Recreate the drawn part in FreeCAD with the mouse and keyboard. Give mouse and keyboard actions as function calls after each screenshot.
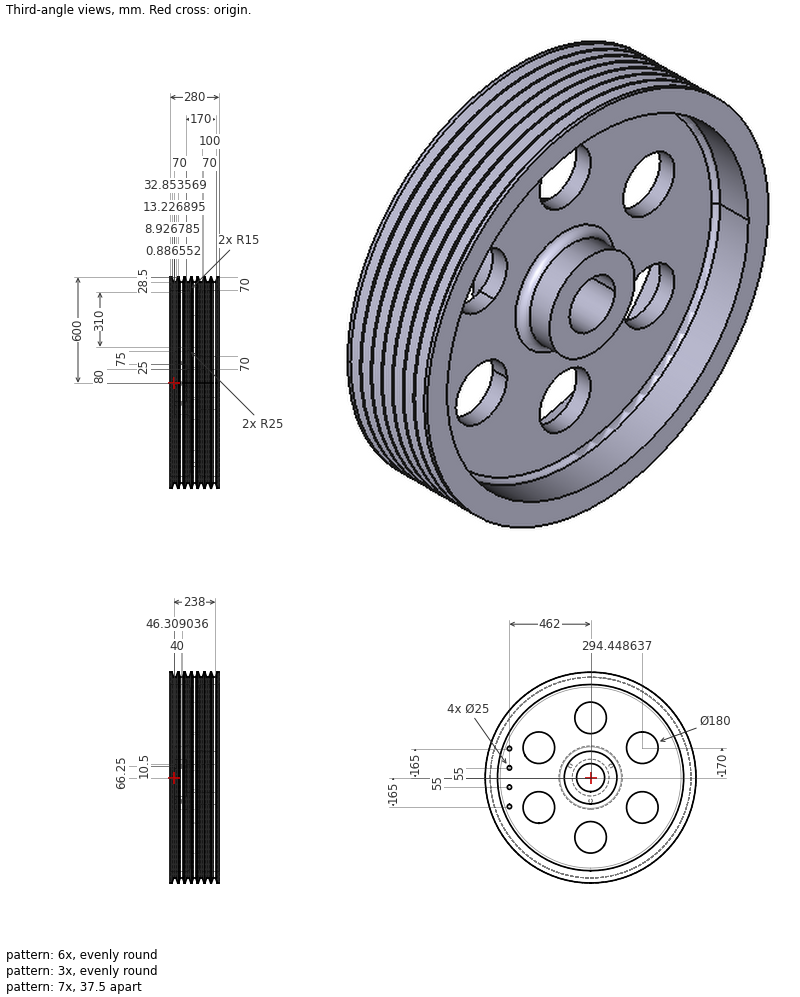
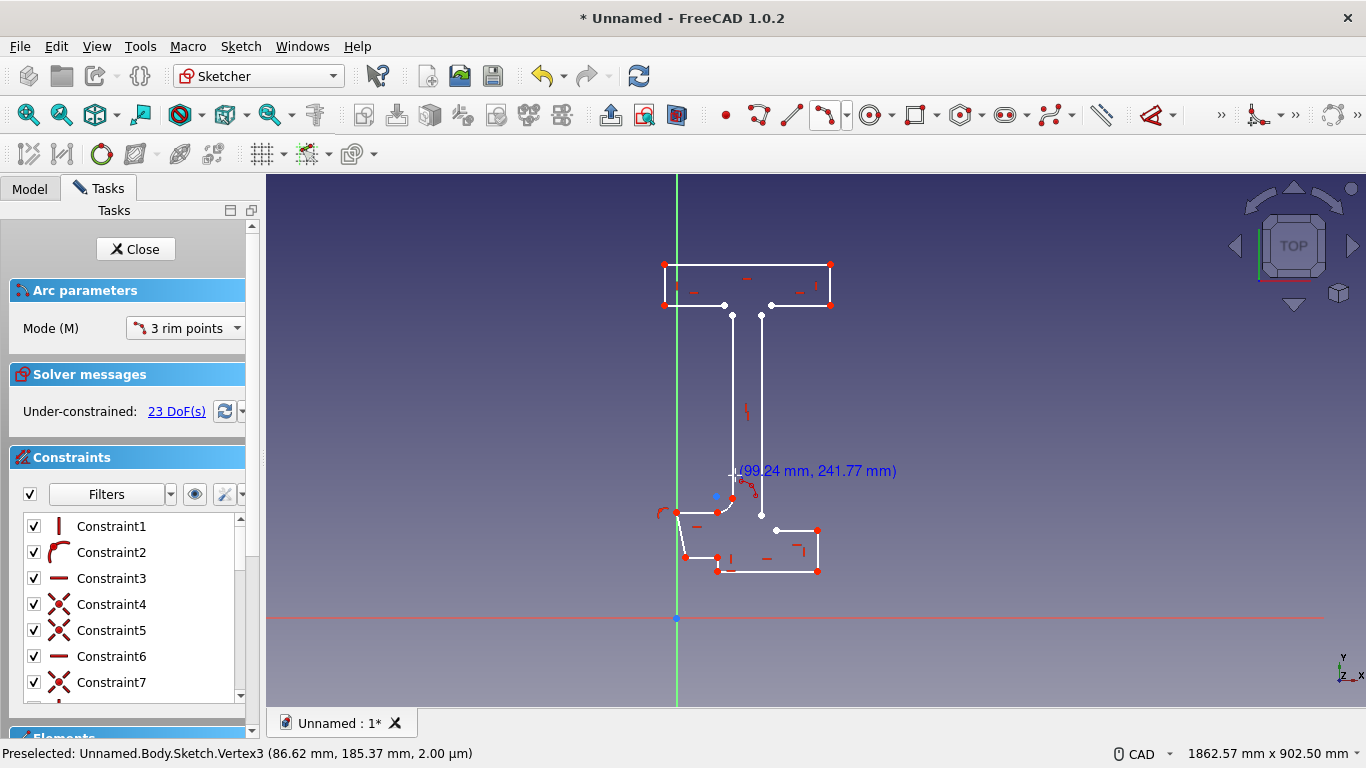
click(777, 531)
click(762, 516)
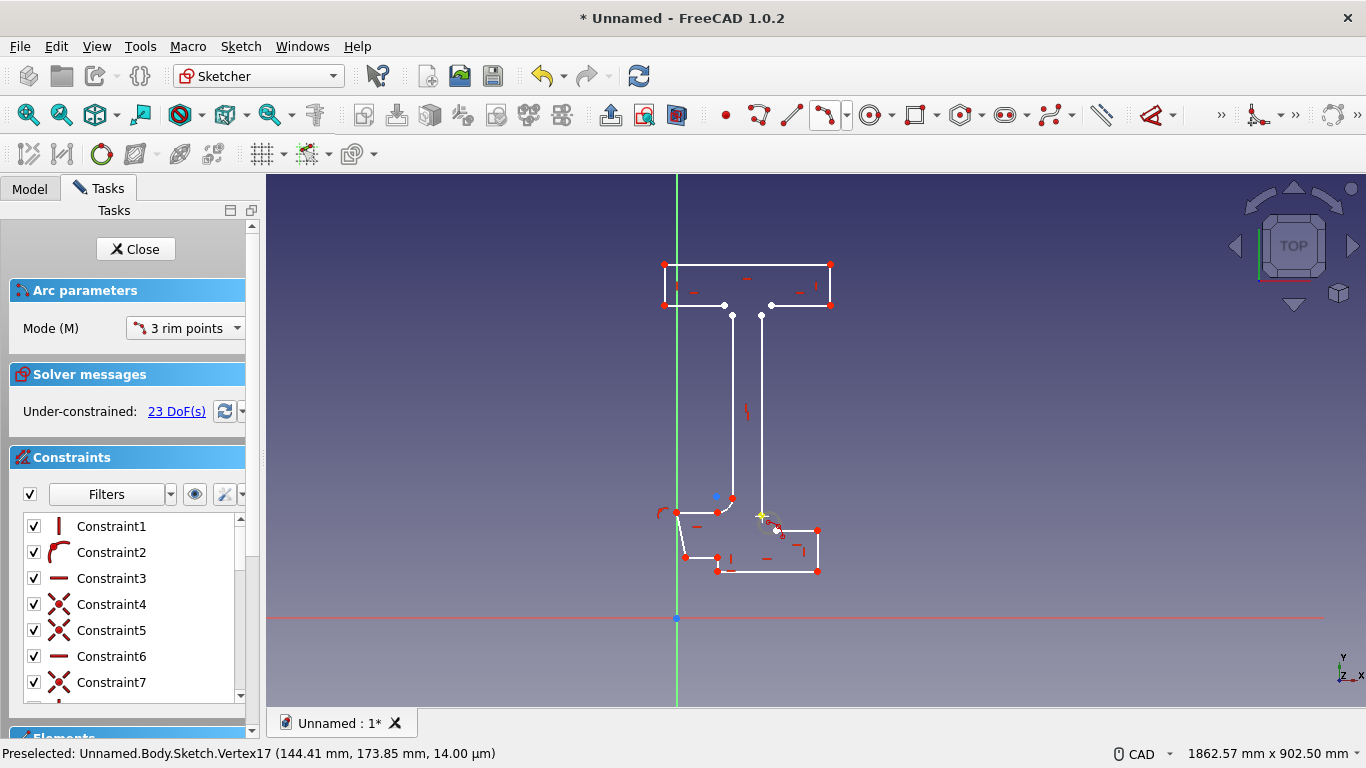
scroll(767, 526, up, 7)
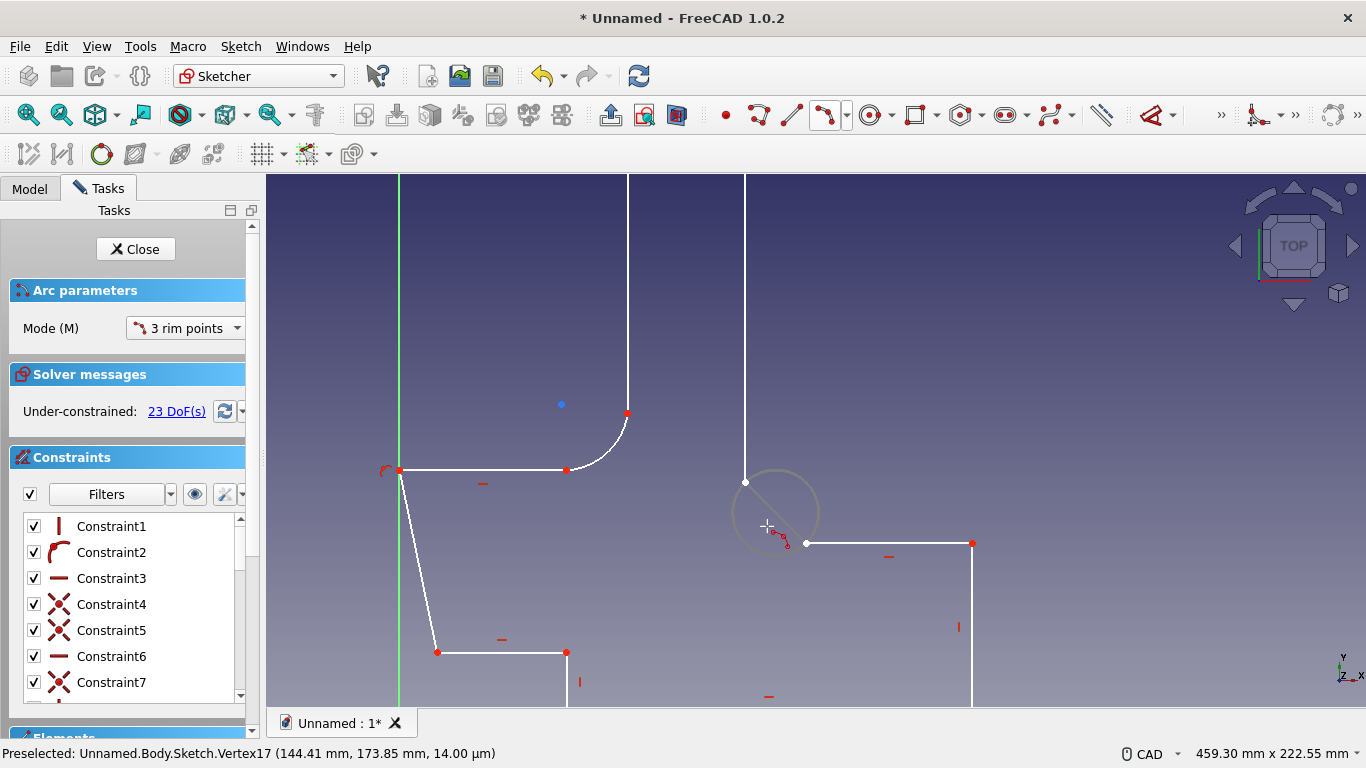
click(764, 522)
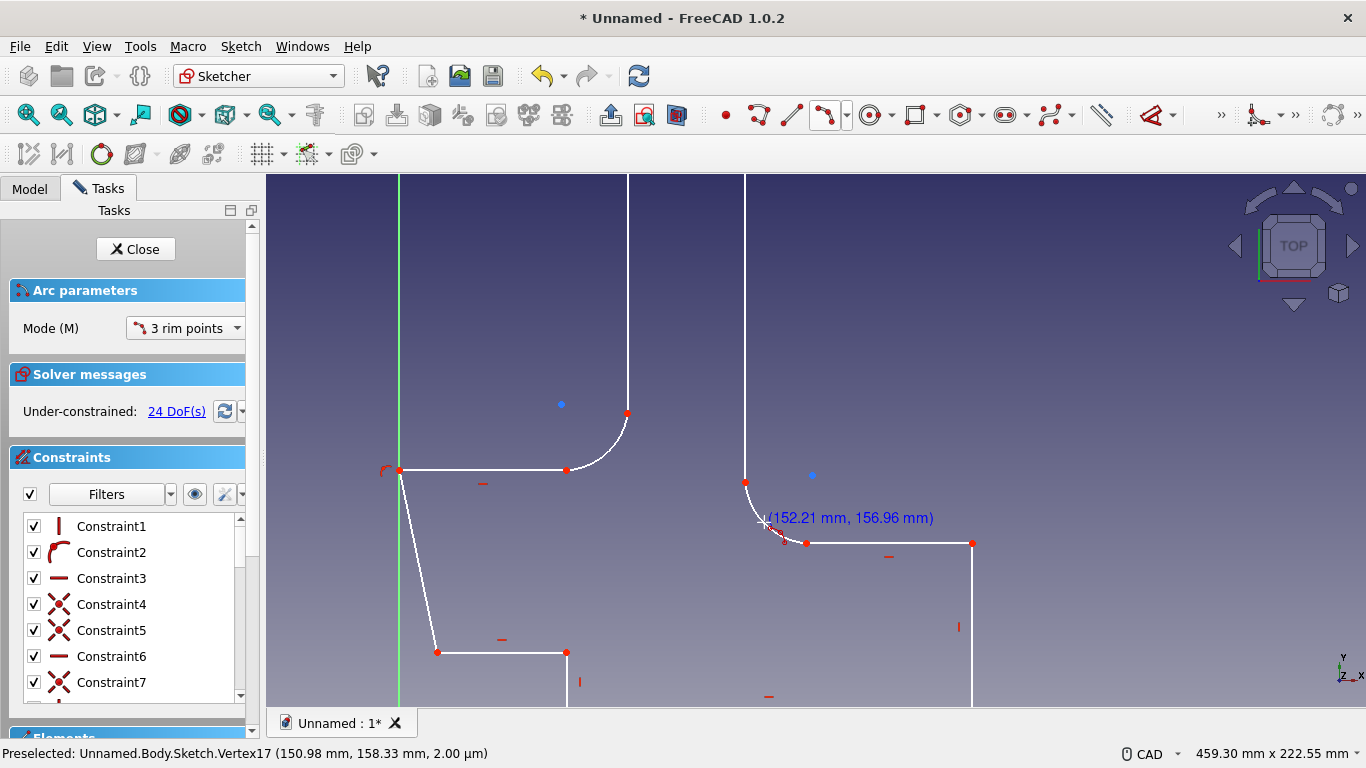
scroll(767, 526, down, 7)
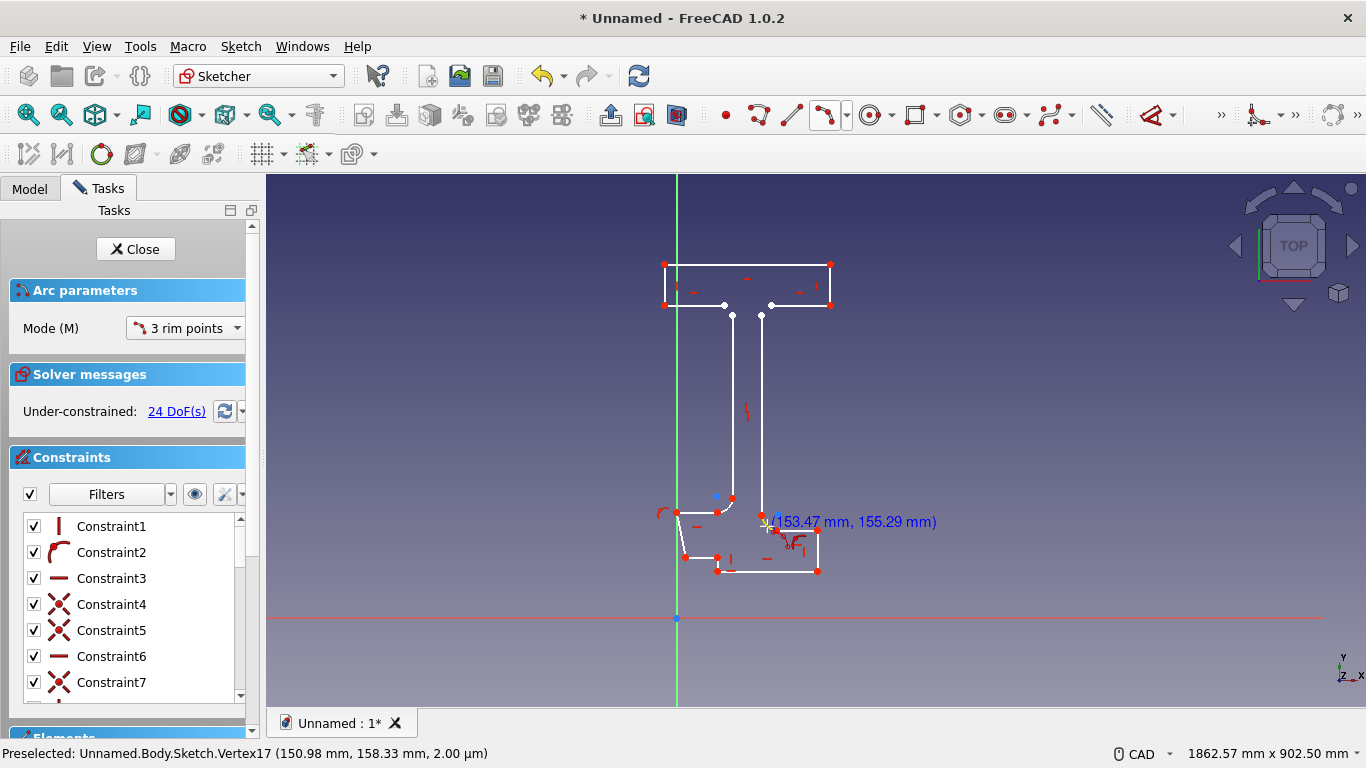
scroll(762, 314, up, 2)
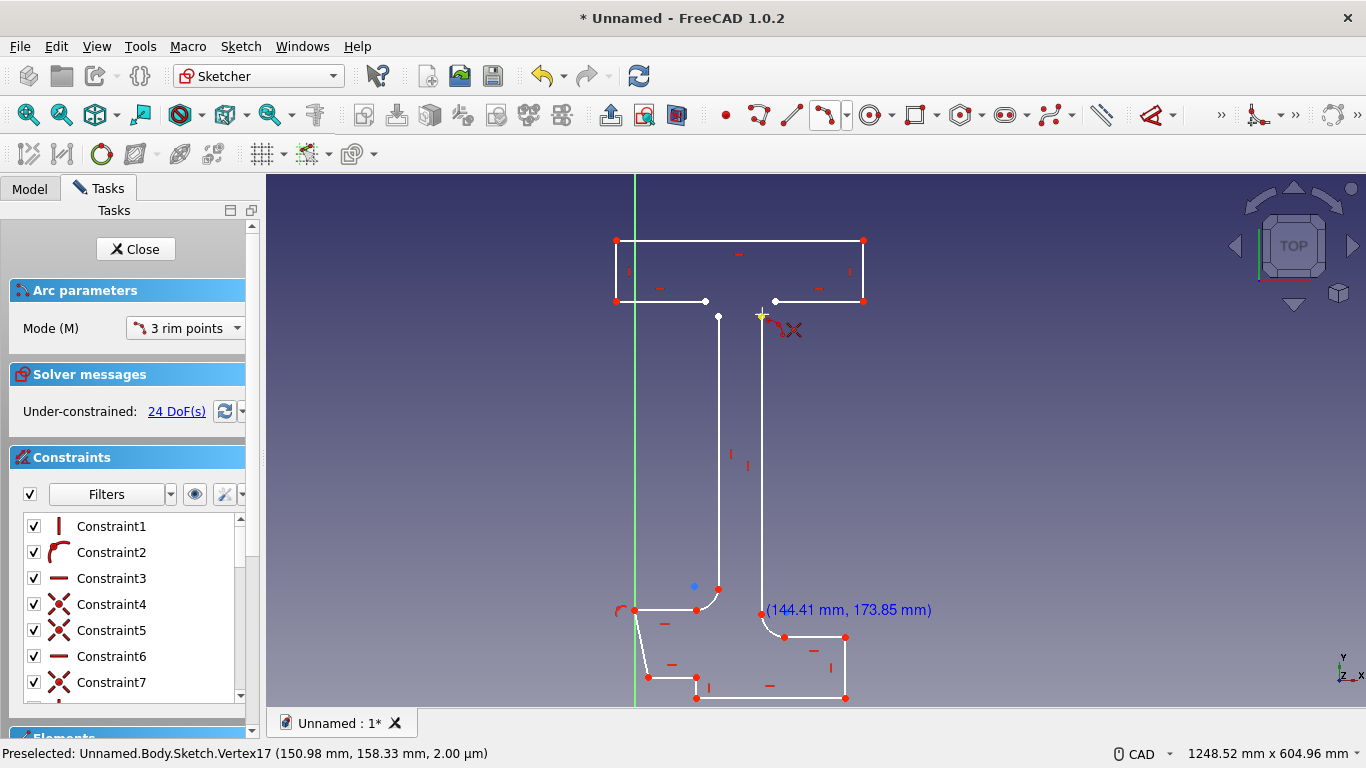
click(762, 317)
click(775, 302)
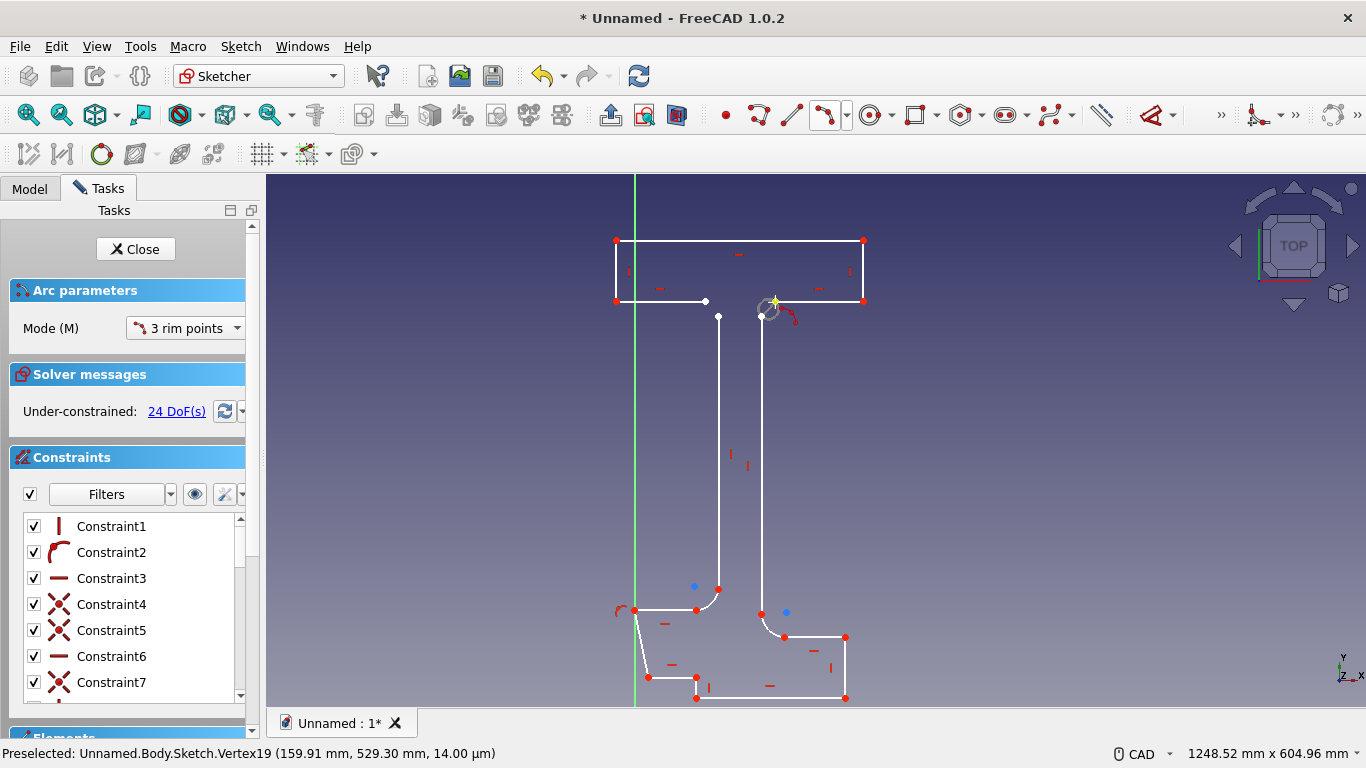
scroll(766, 305, up, 8)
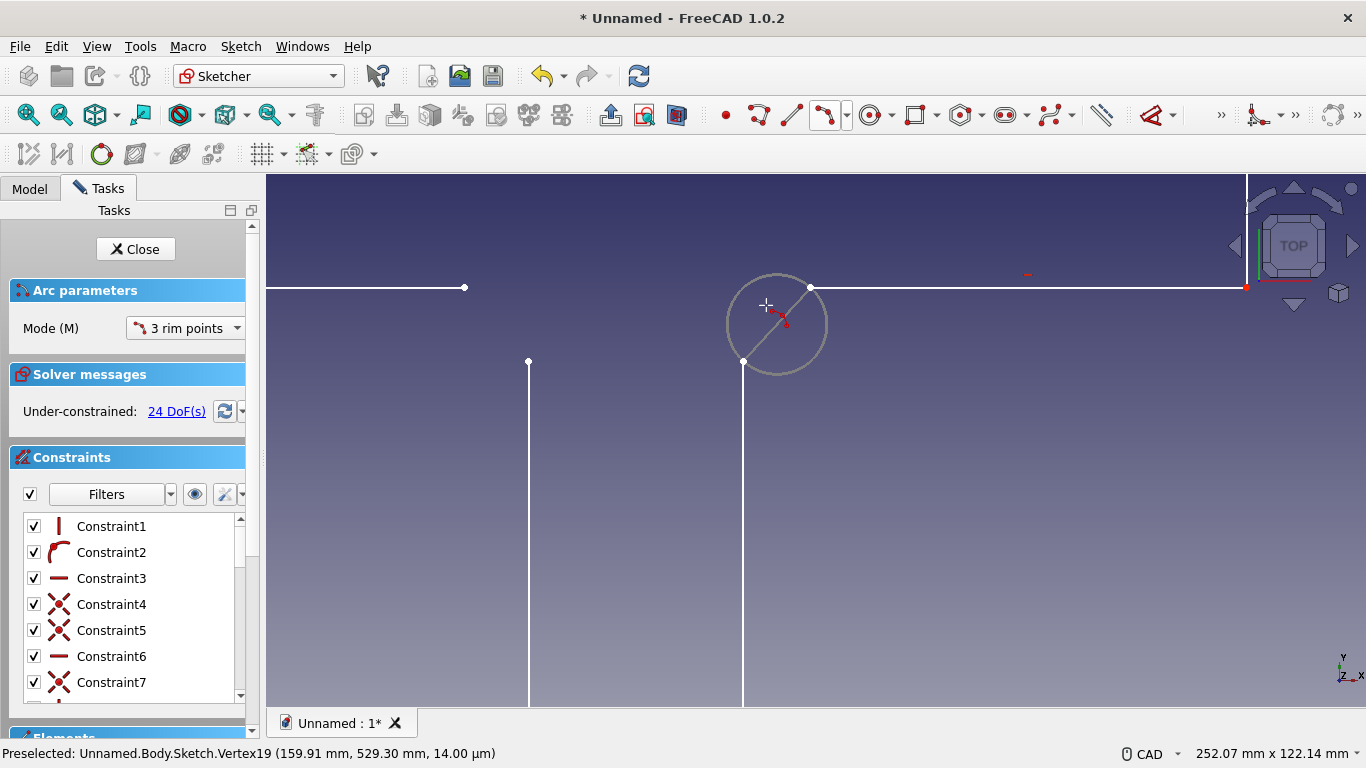
click(765, 304)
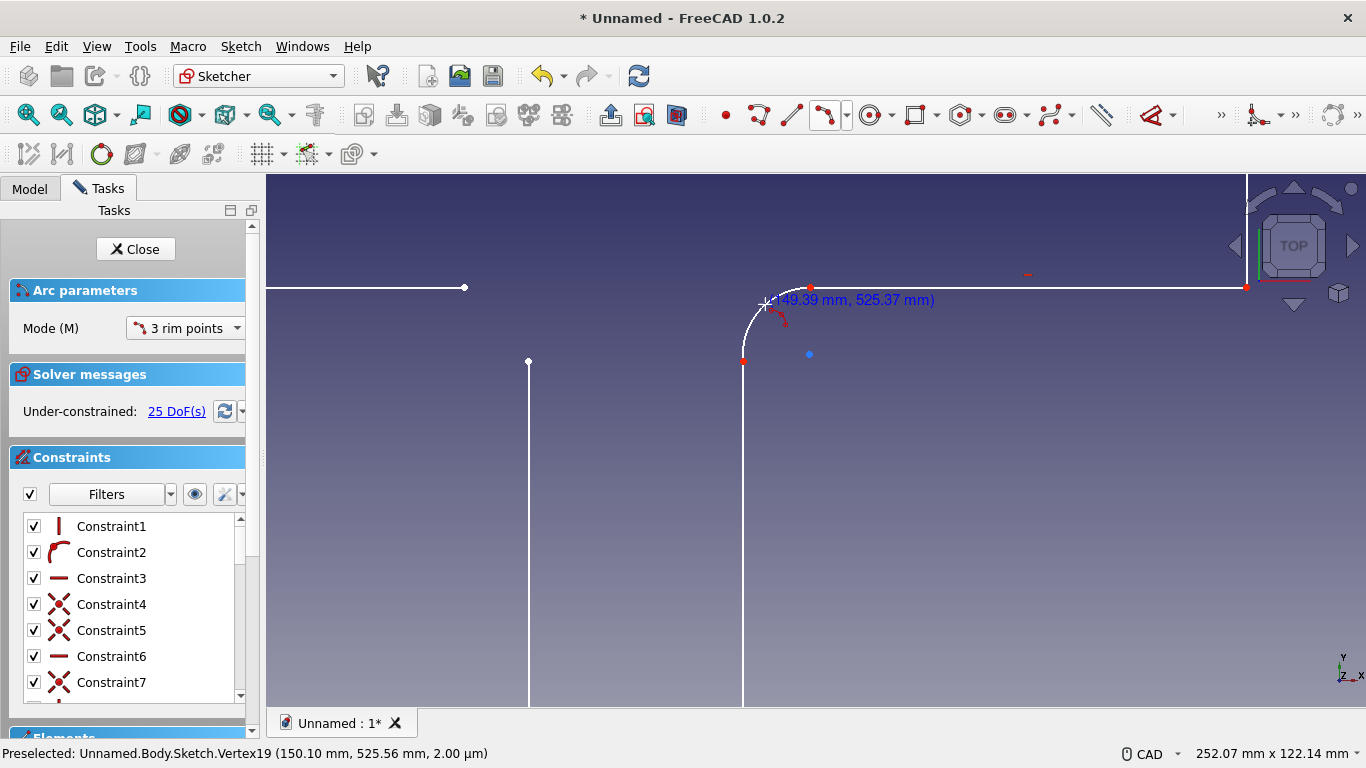
scroll(765, 308, down, 10)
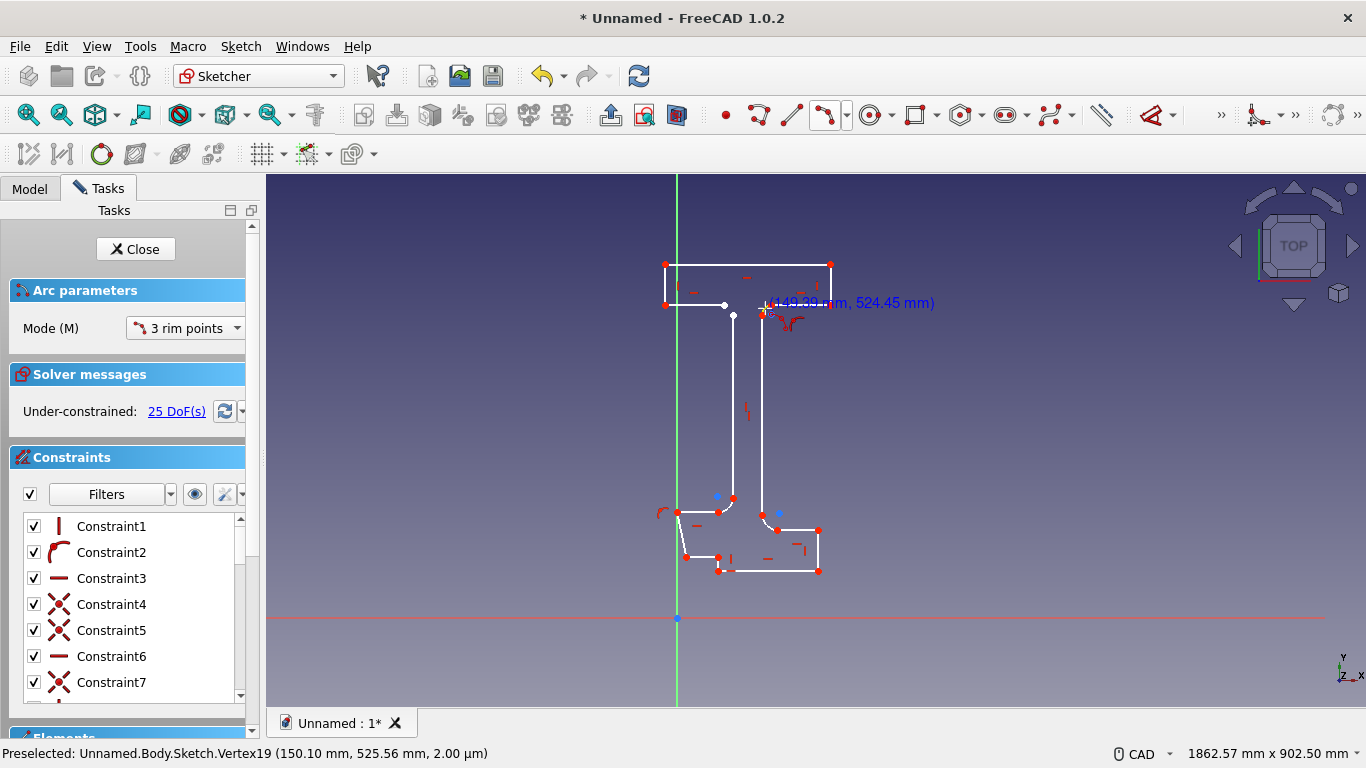
scroll(724, 305, up, 2)